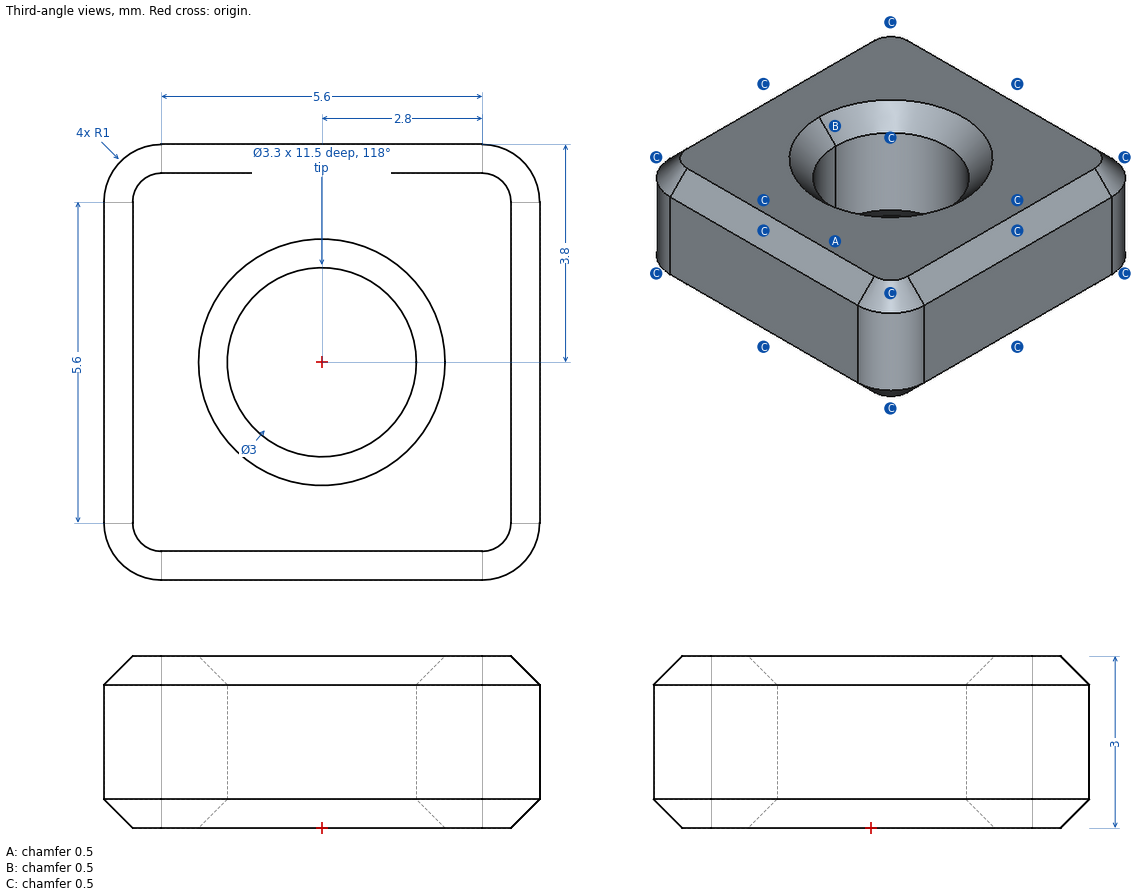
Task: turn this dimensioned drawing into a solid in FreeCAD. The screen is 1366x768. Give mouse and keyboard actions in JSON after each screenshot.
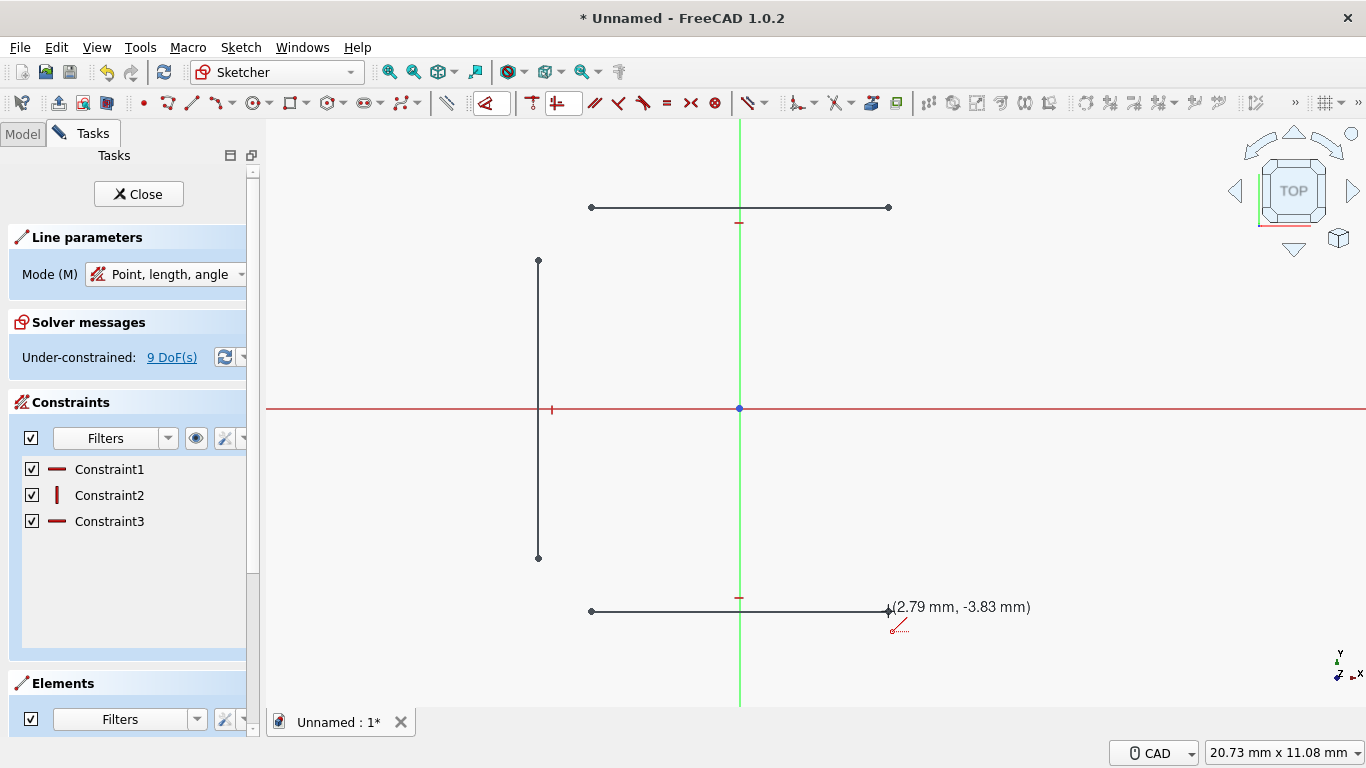
{"action": "left_click", "coordinate": [941, 558]}
{"action": "left_click", "coordinate": [941, 260]}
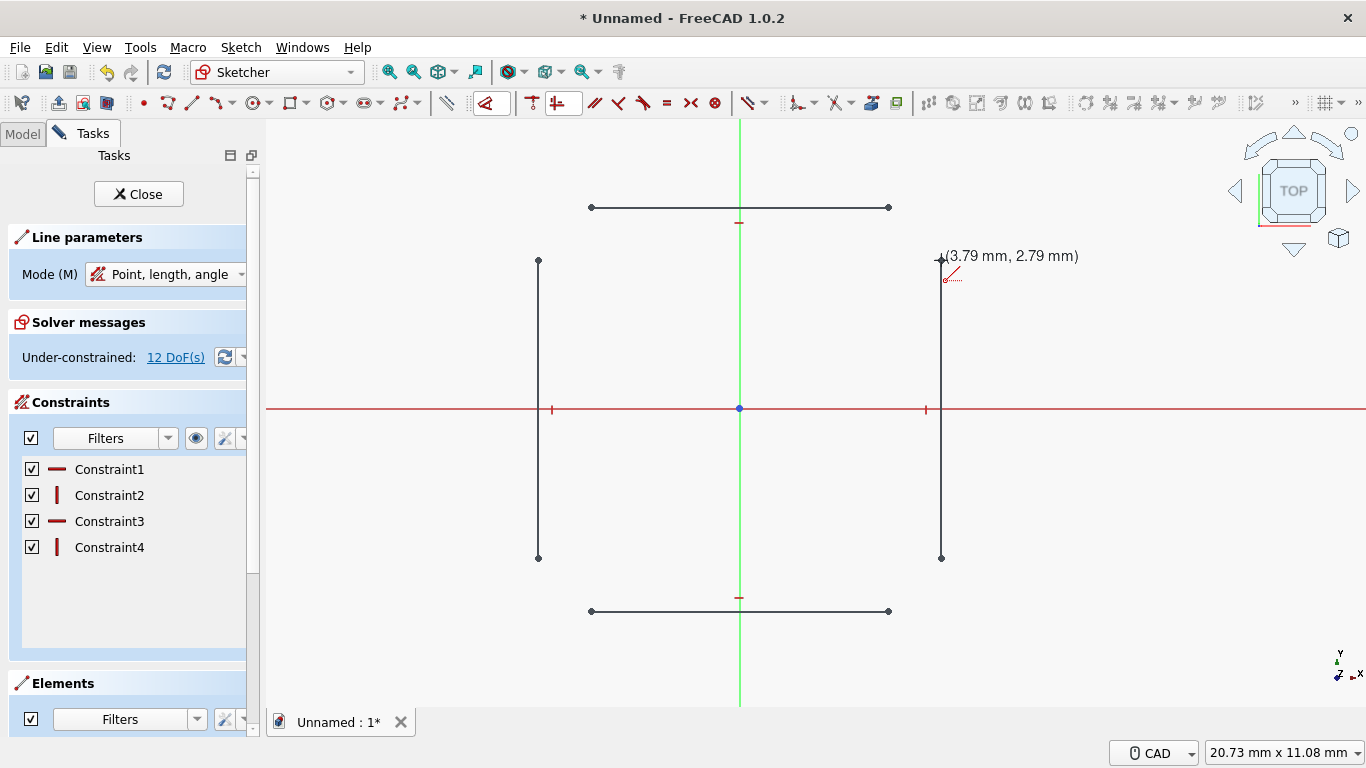
{"action": "key", "text": "g 3 a"}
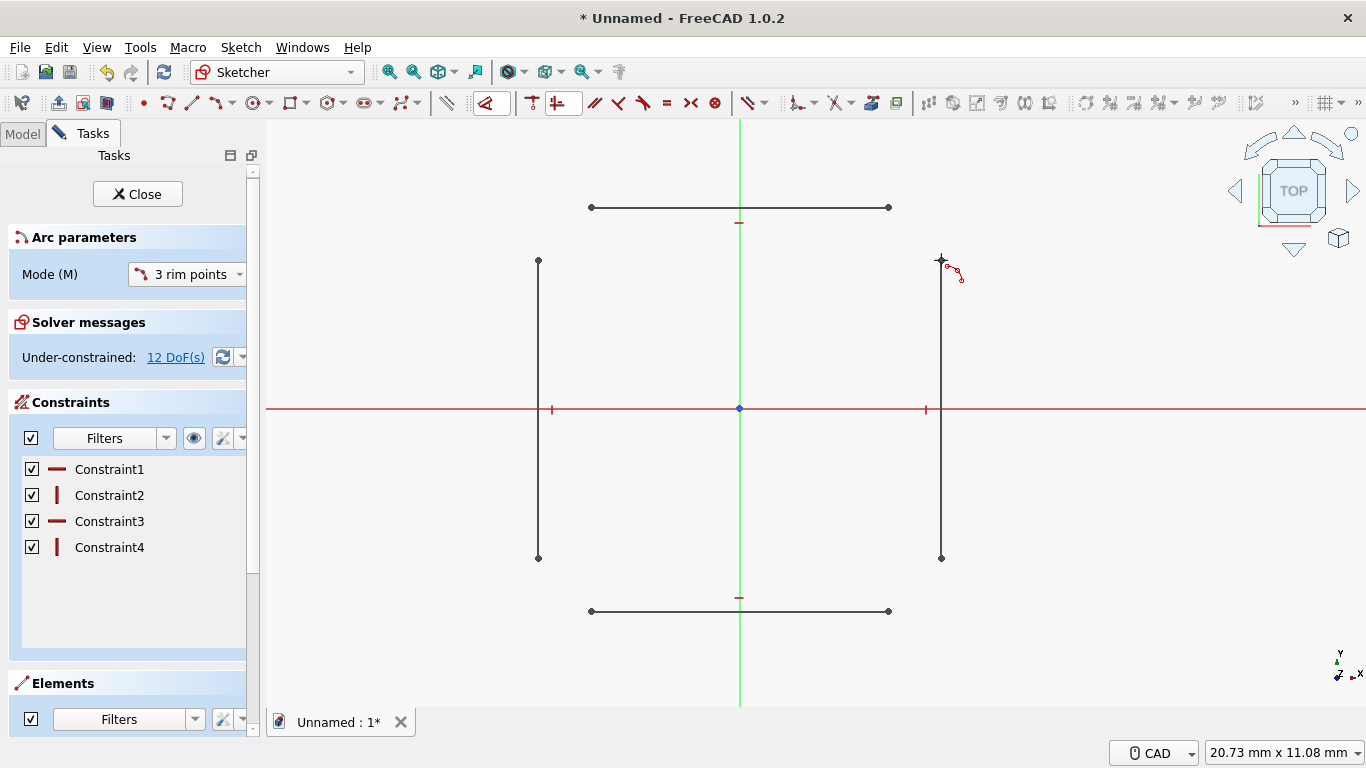
{"action": "left_click", "coordinate": [591, 208]}
{"action": "left_click", "coordinate": [538, 261]}
{"action": "left_click", "coordinate": [554, 223]}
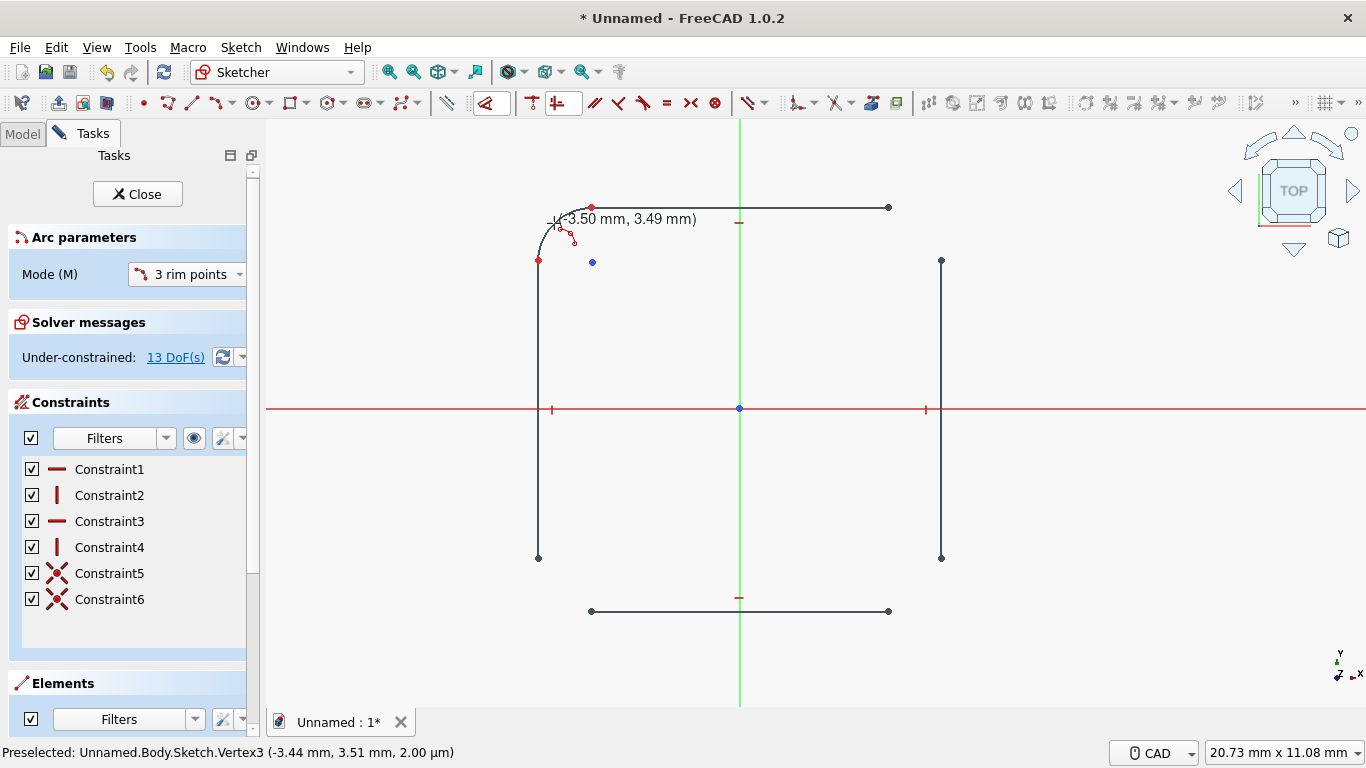
{"action": "left_click", "coordinate": [538, 559]}
{"action": "left_click", "coordinate": [591, 612]}
{"action": "left_click", "coordinate": [554, 595]}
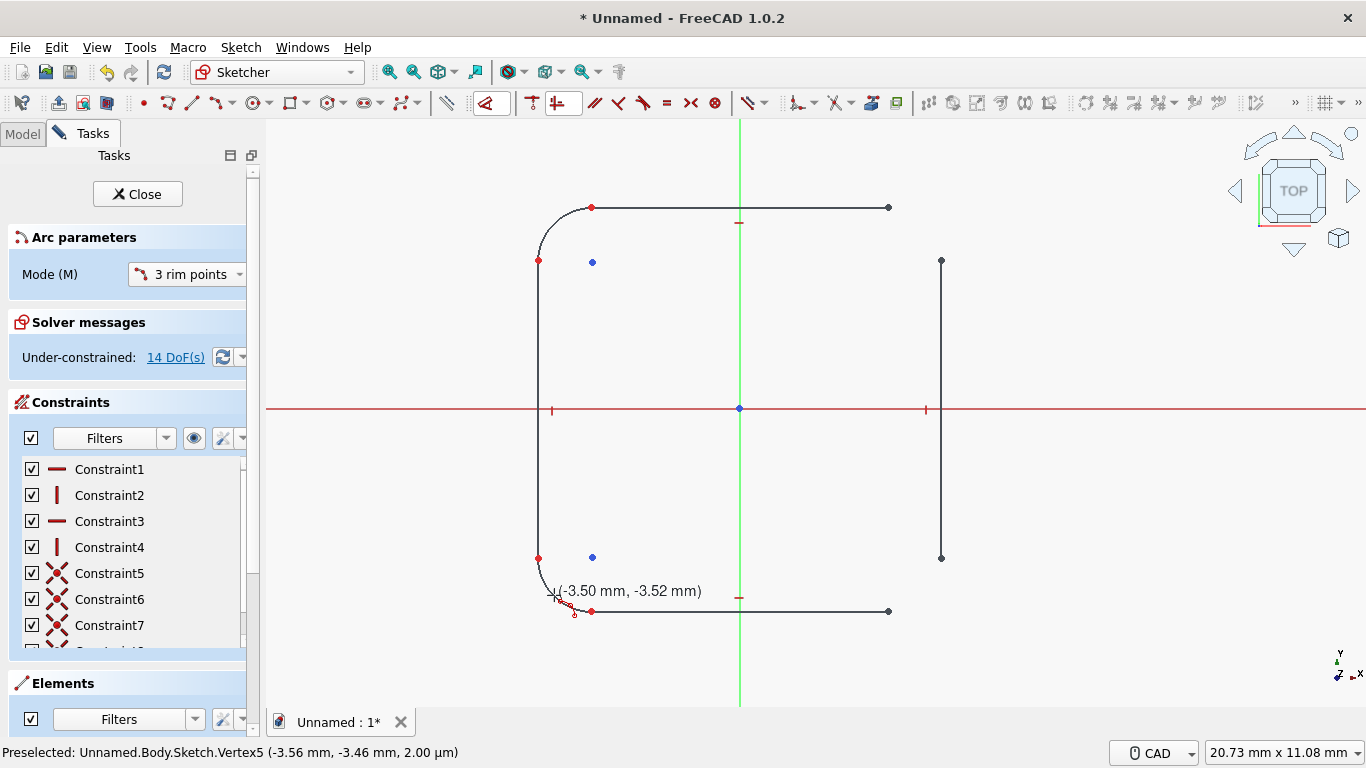
{"action": "left_click", "coordinate": [888, 612]}
{"action": "left_click", "coordinate": [941, 559]}
{"action": "left_click", "coordinate": [926, 595]}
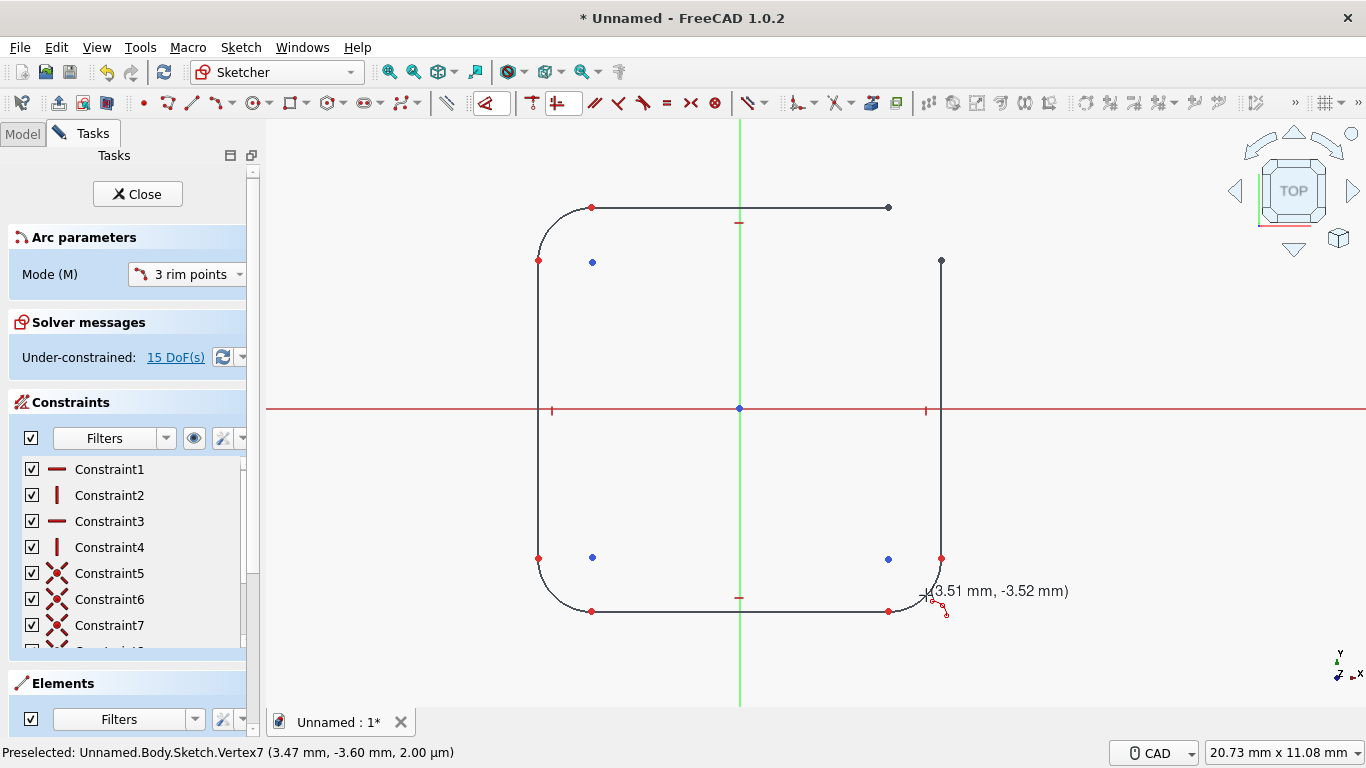
{"action": "left_click", "coordinate": [941, 261]}
{"action": "left_click", "coordinate": [888, 208]}
{"action": "left_click", "coordinate": [926, 223]}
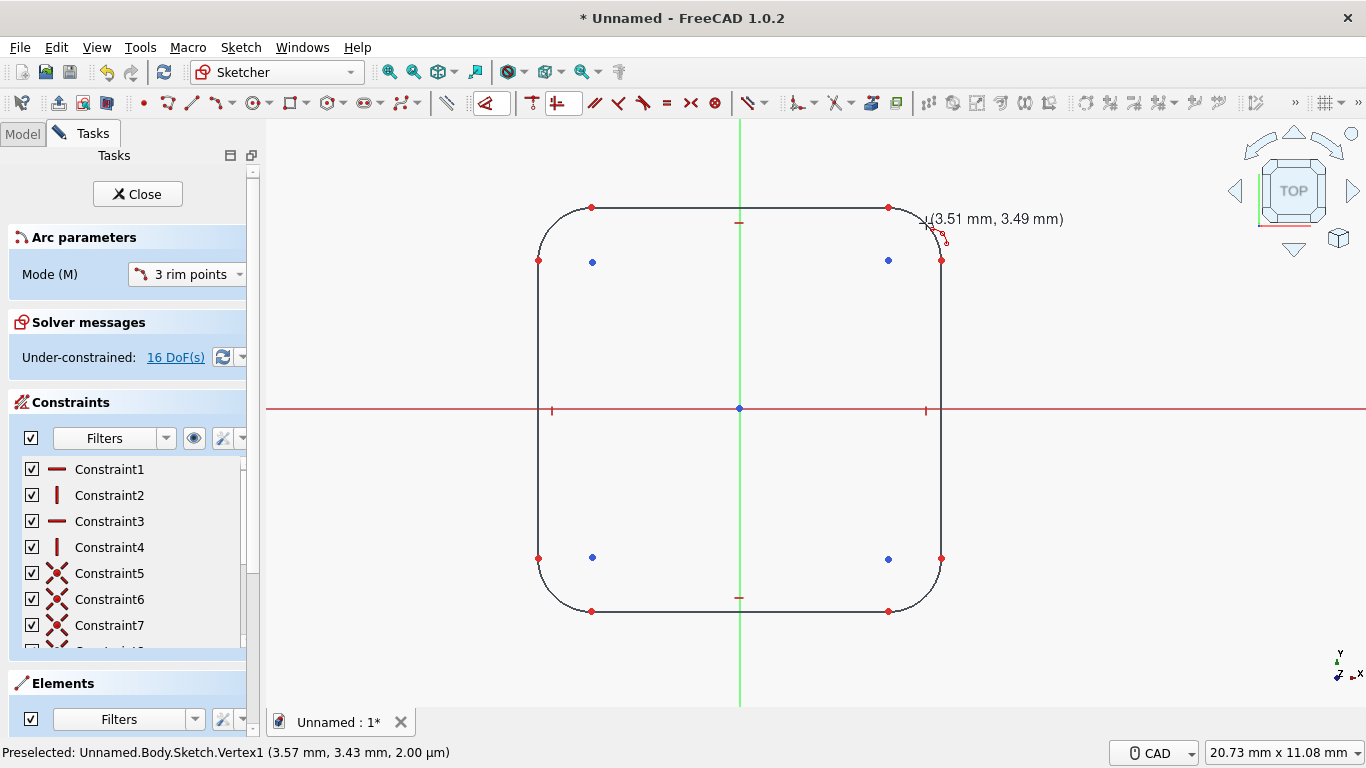
{"action": "key", "text": "g c"}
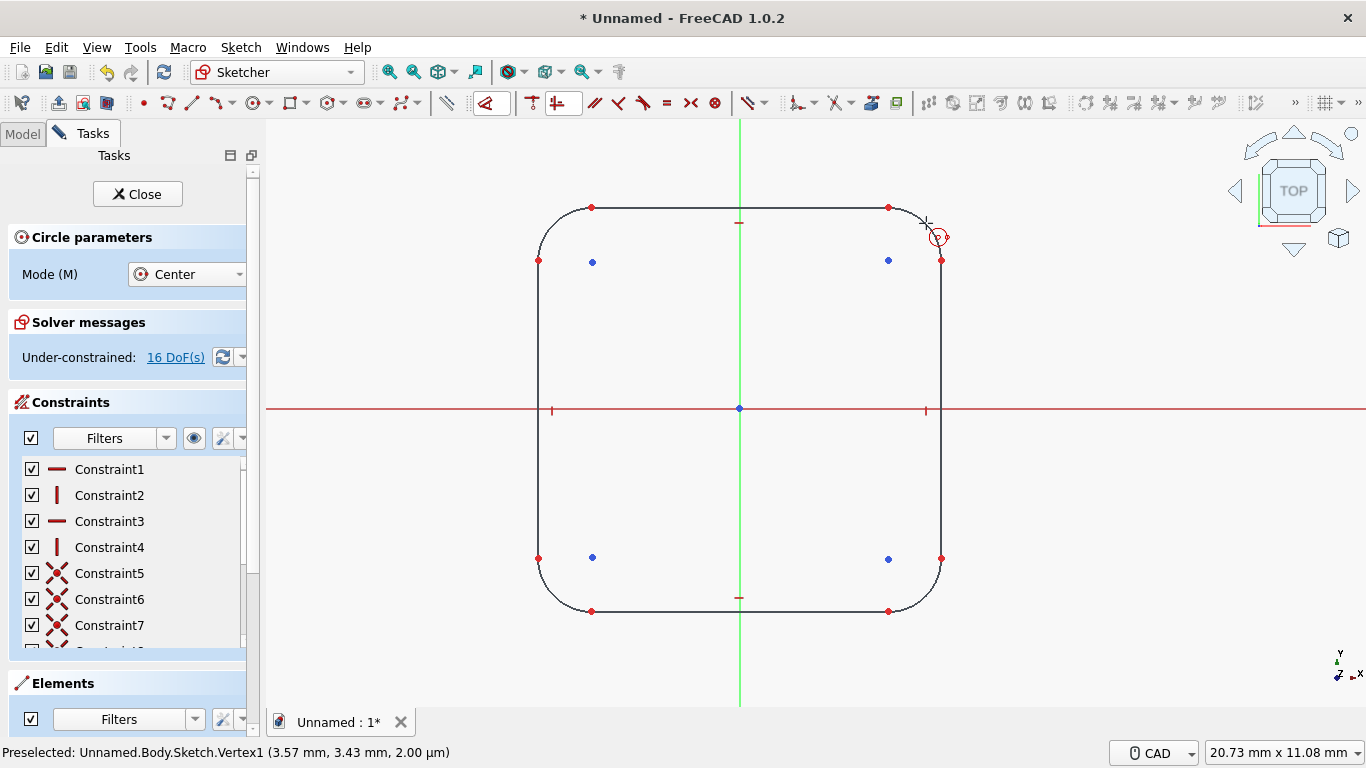
{"action": "left_click", "coordinate": [740, 409]}
{"action": "left_click", "coordinate": [796, 353]}
{"action": "key", "text": "Escape"}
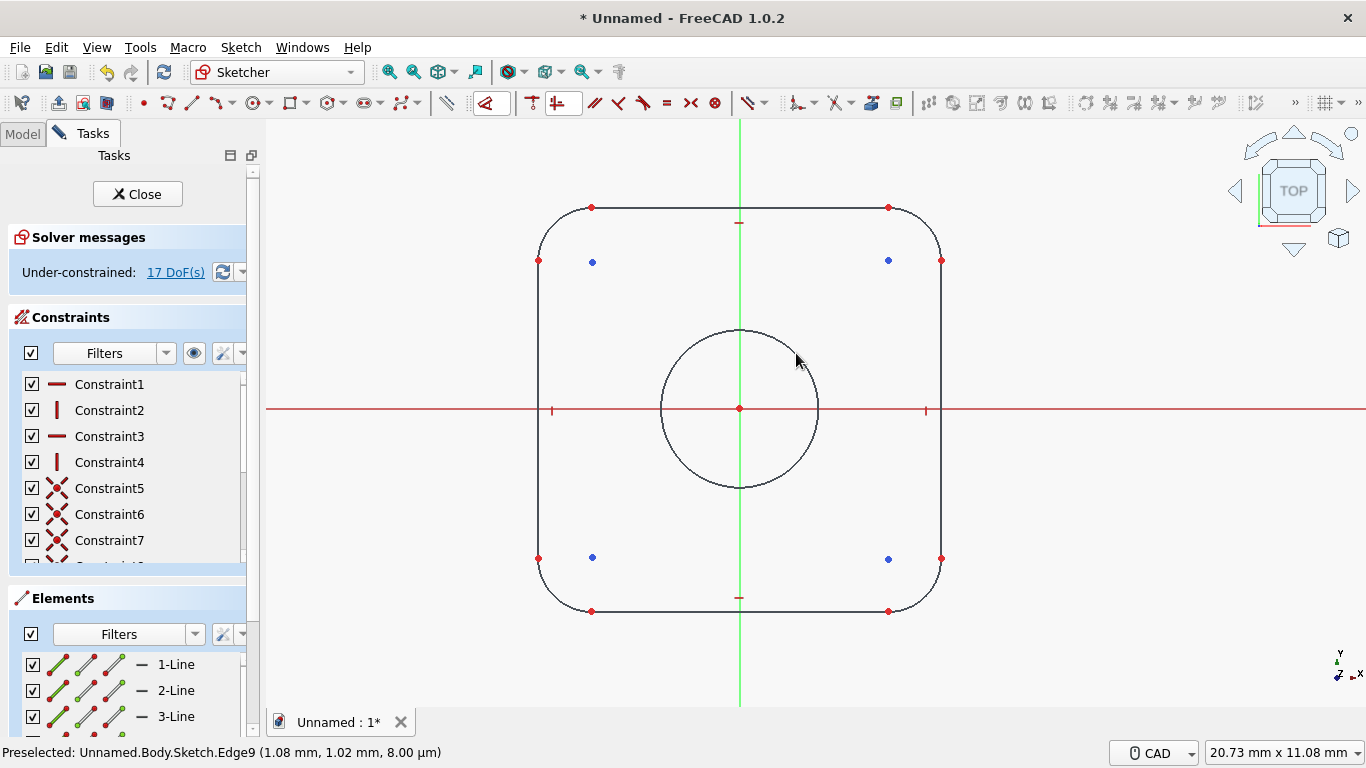
{"action": "left_click", "coordinate": [799, 208]}